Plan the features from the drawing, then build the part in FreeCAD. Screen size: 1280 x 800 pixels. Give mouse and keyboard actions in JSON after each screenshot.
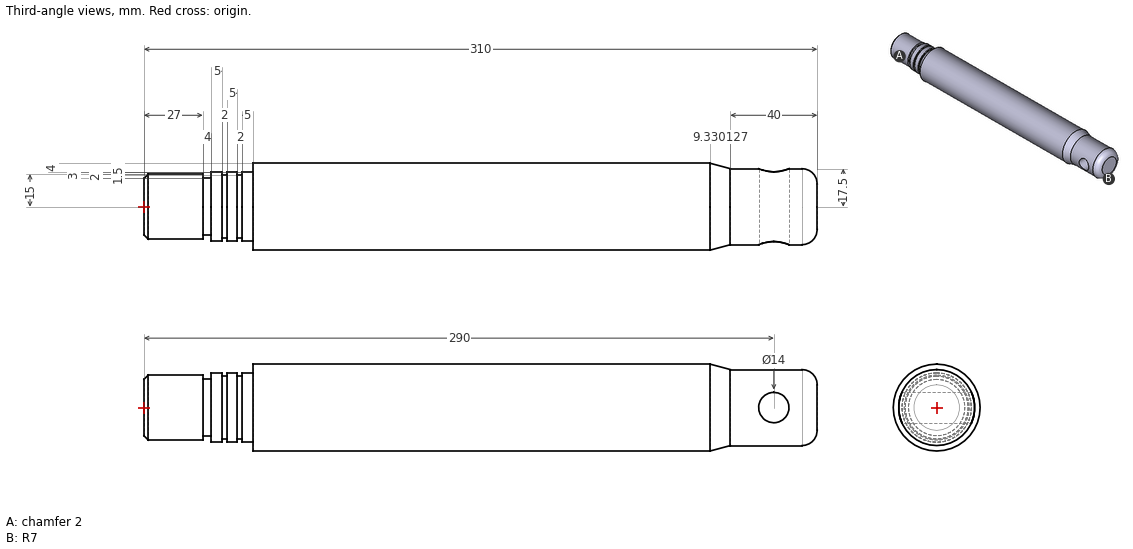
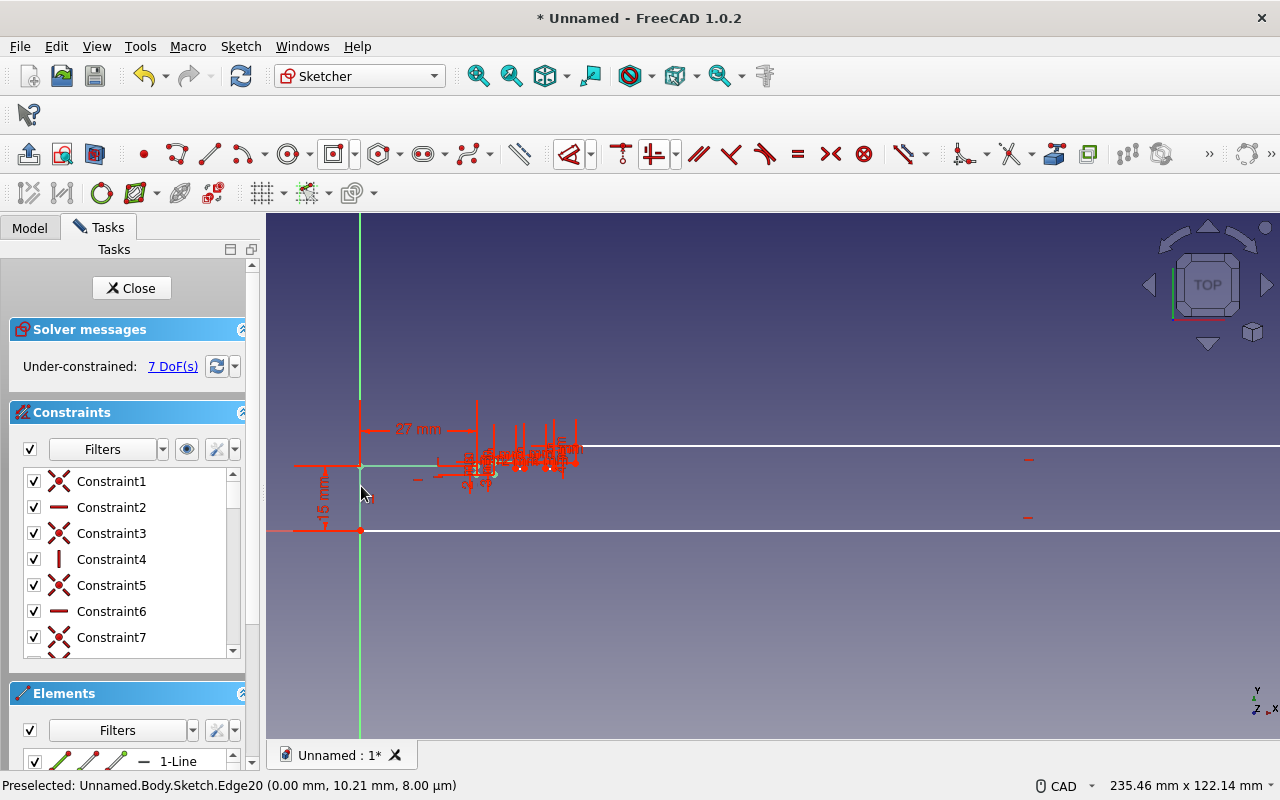
{"action": "left_click", "coordinate": [761, 531]}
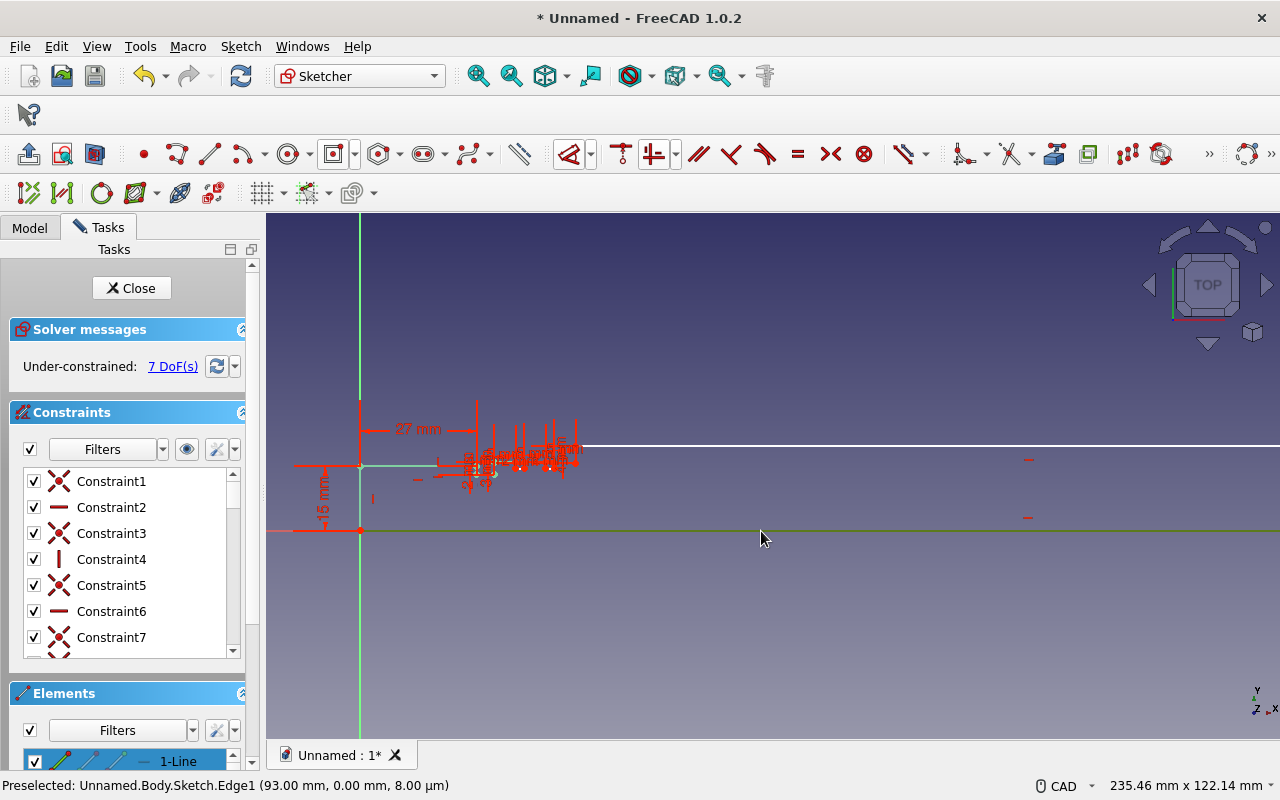
{"action": "left_click", "coordinate": [590, 154]}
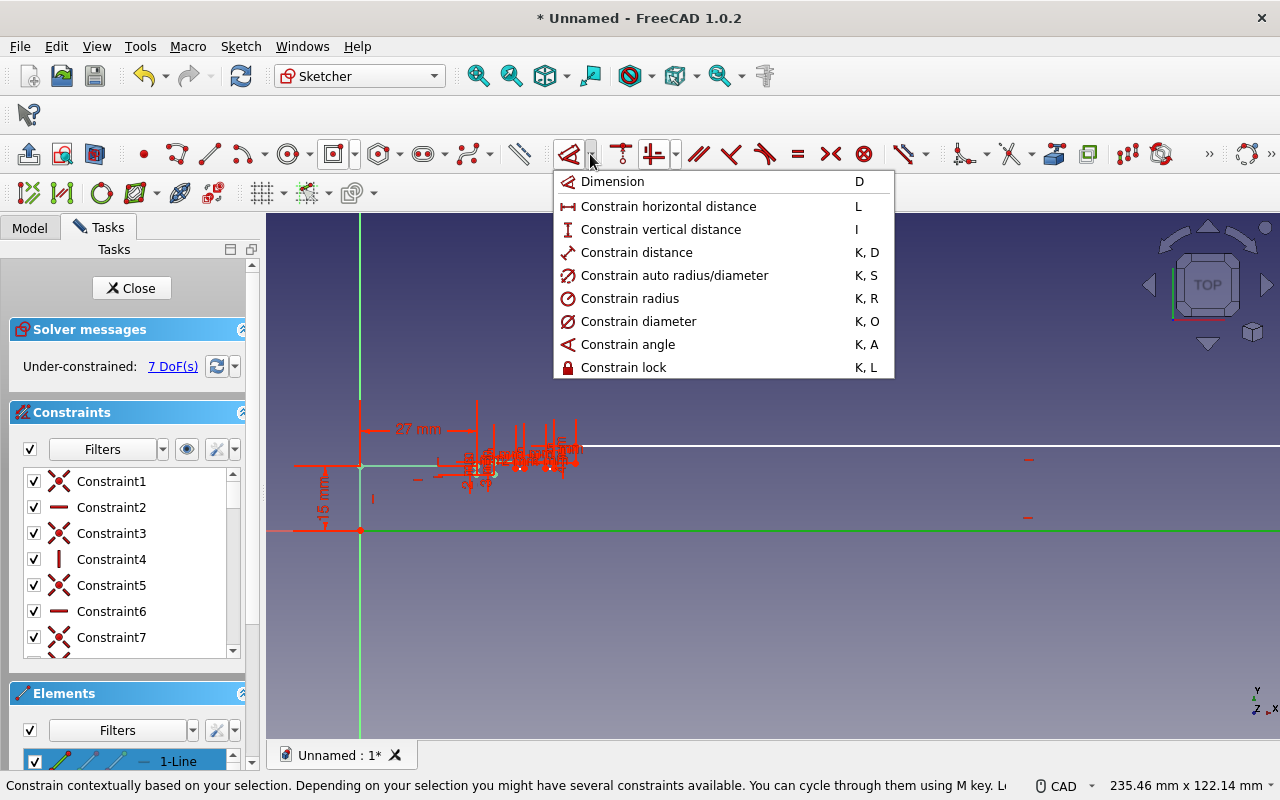
{"action": "left_click", "coordinate": [724, 206]}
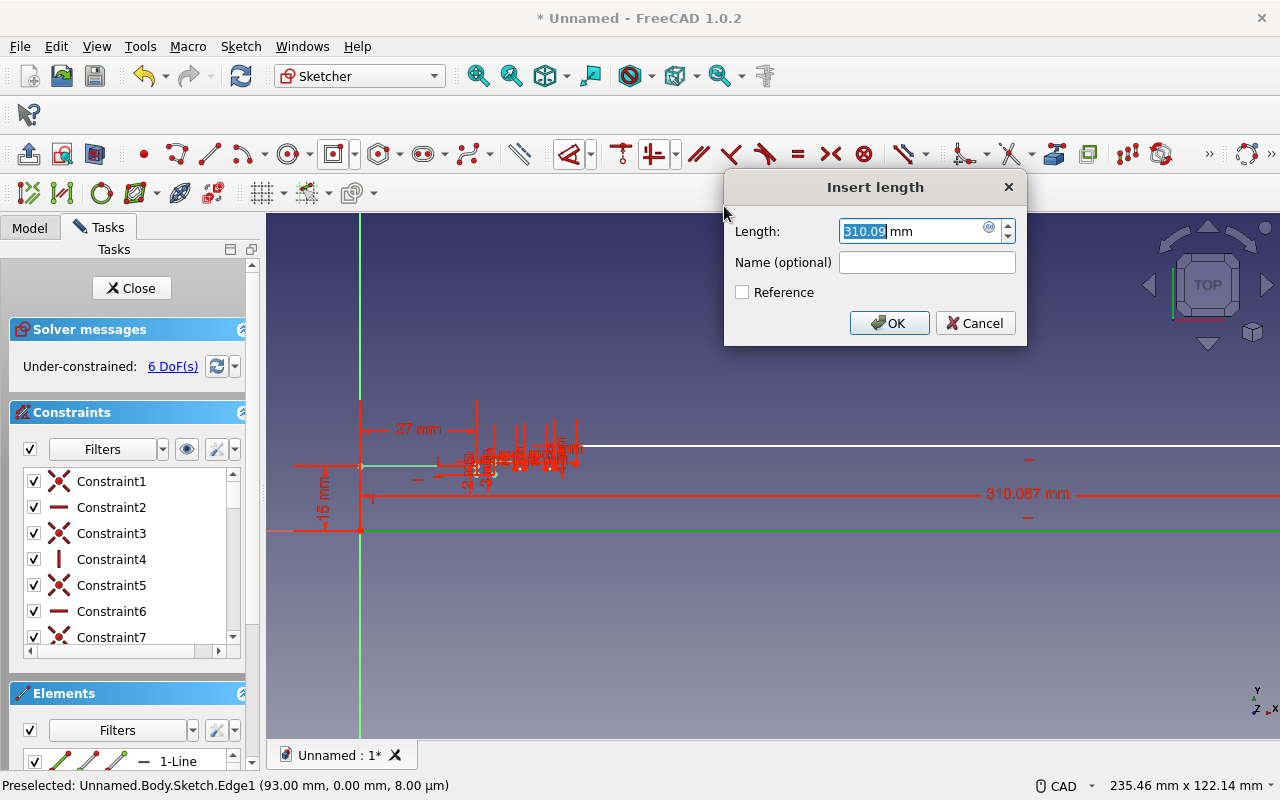
{"action": "type", "text": "310"}
{"action": "key", "text": "Return"}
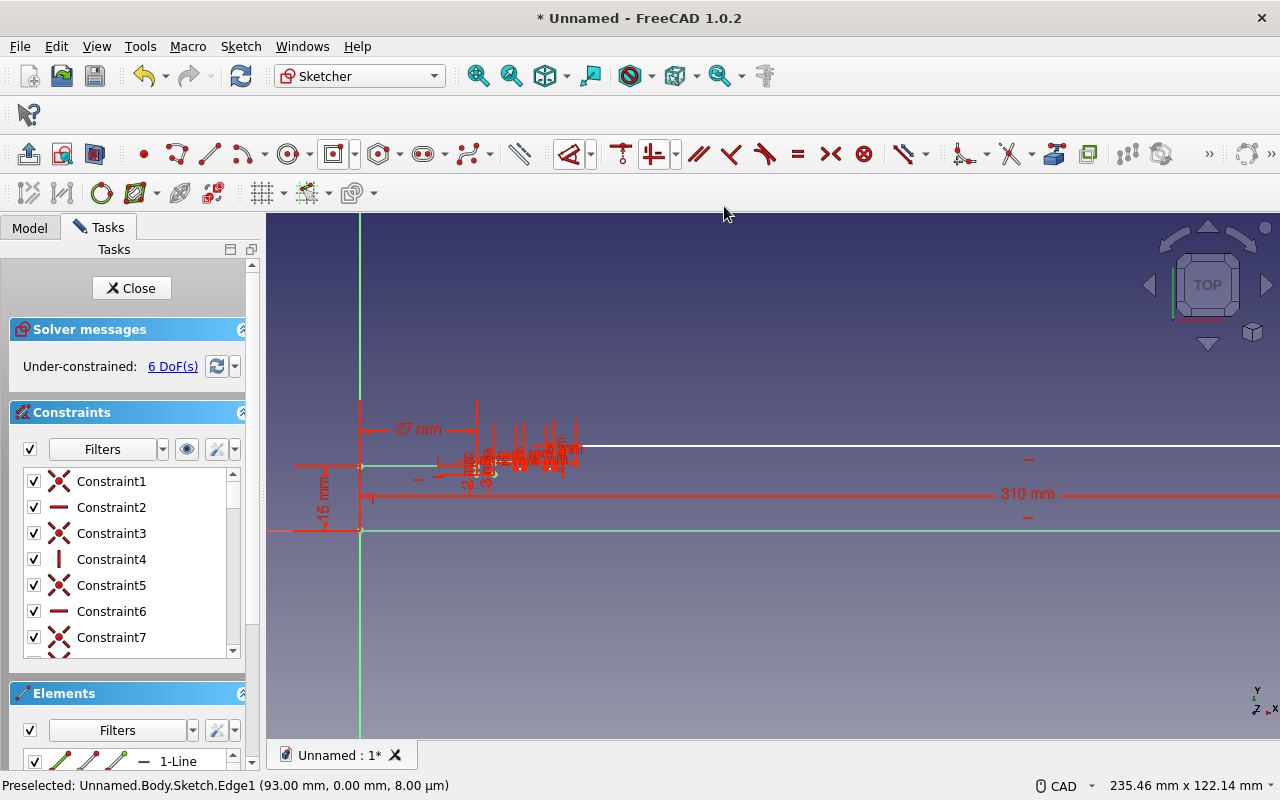
{"action": "scroll", "coordinate": [554, 466], "scroll_direction": "up", "scroll_amount": 10}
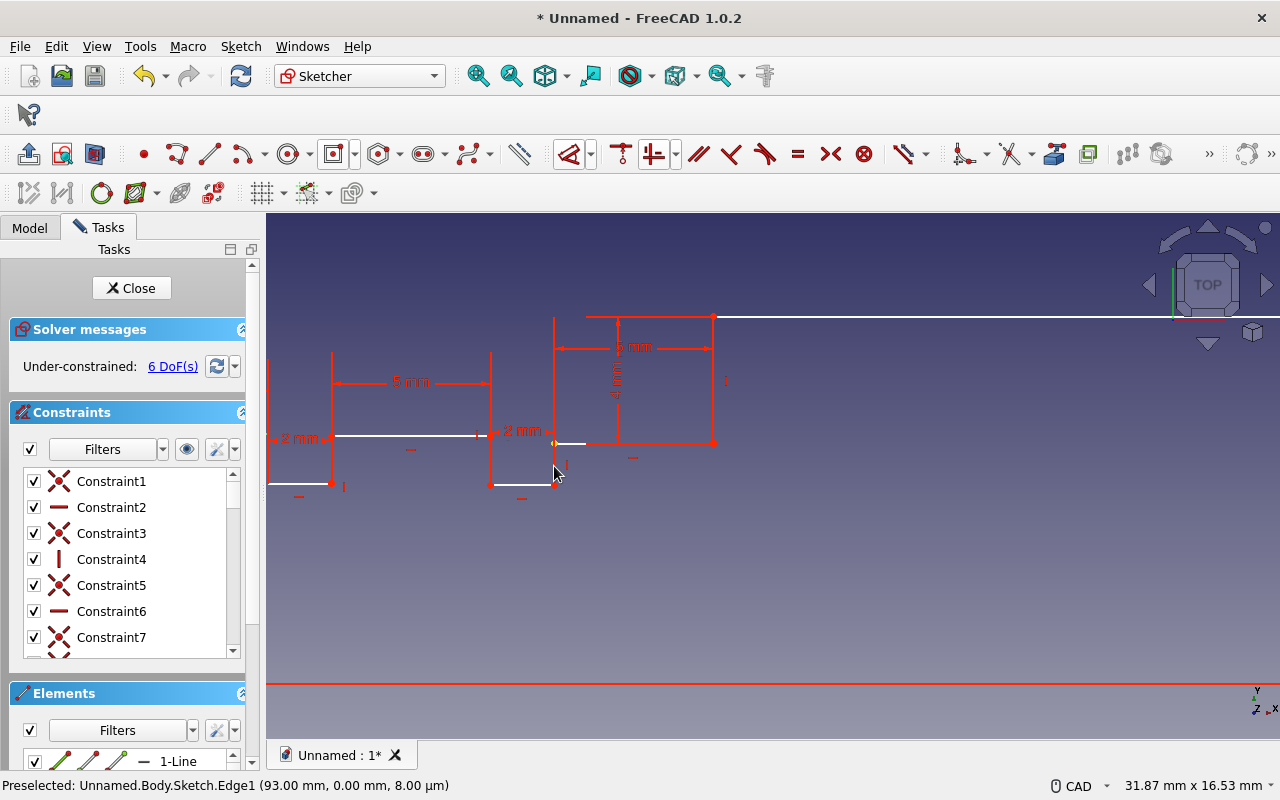
{"action": "left_click", "coordinate": [554, 464]}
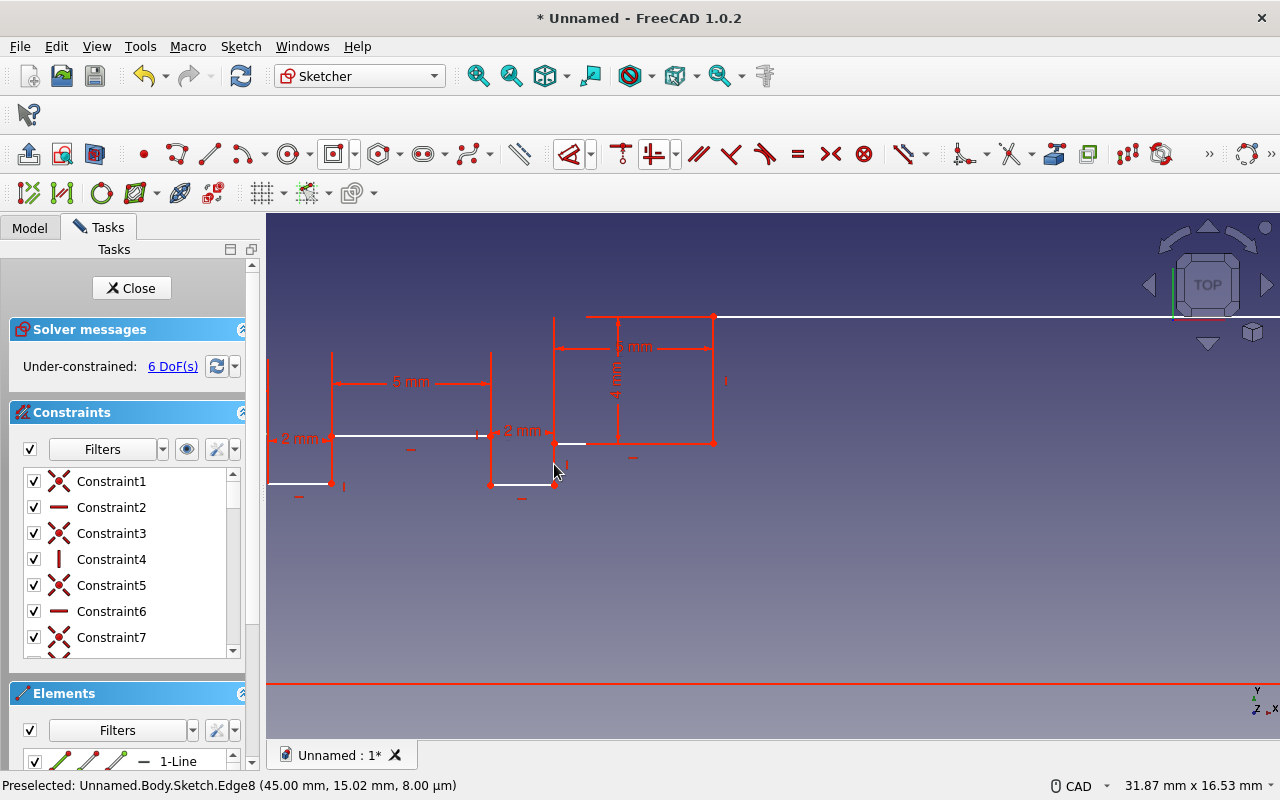
{"action": "key", "text": "i"}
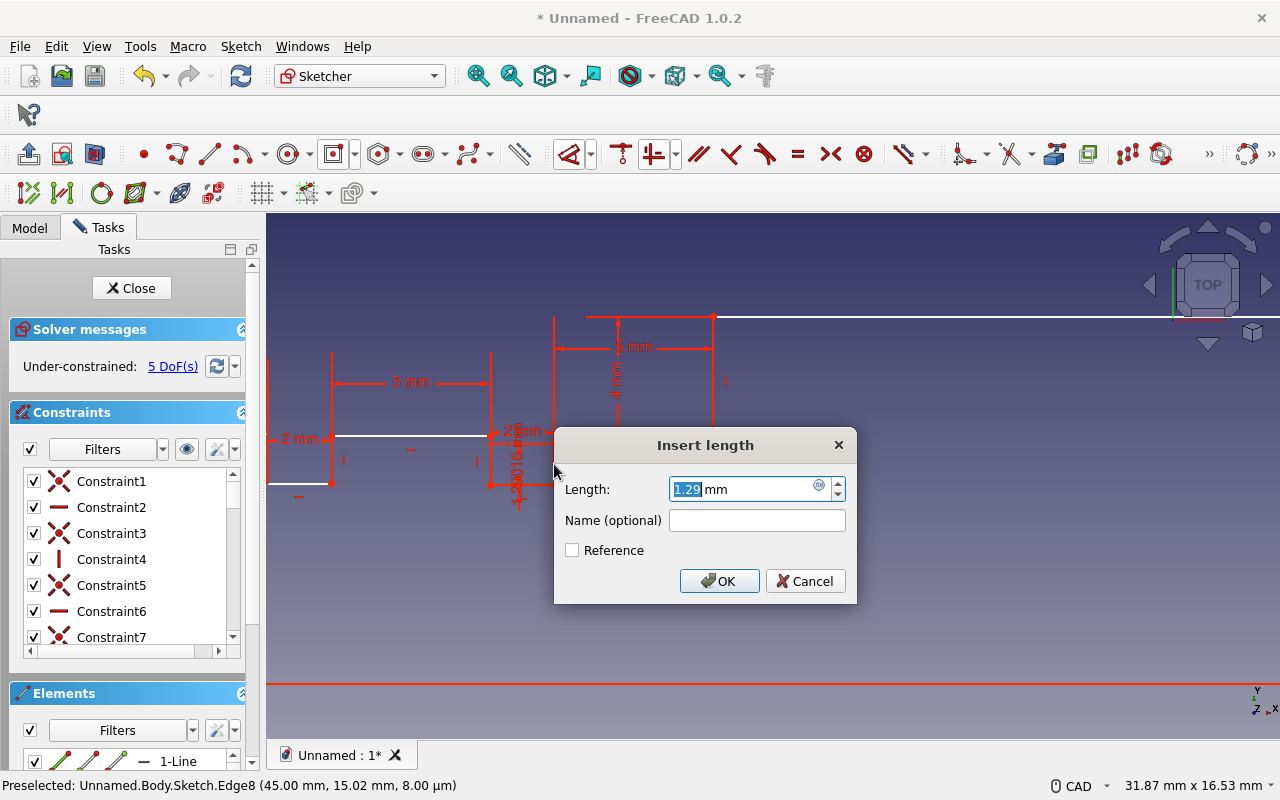
{"action": "type", "text": "1.5"}
{"action": "key", "text": "Return"}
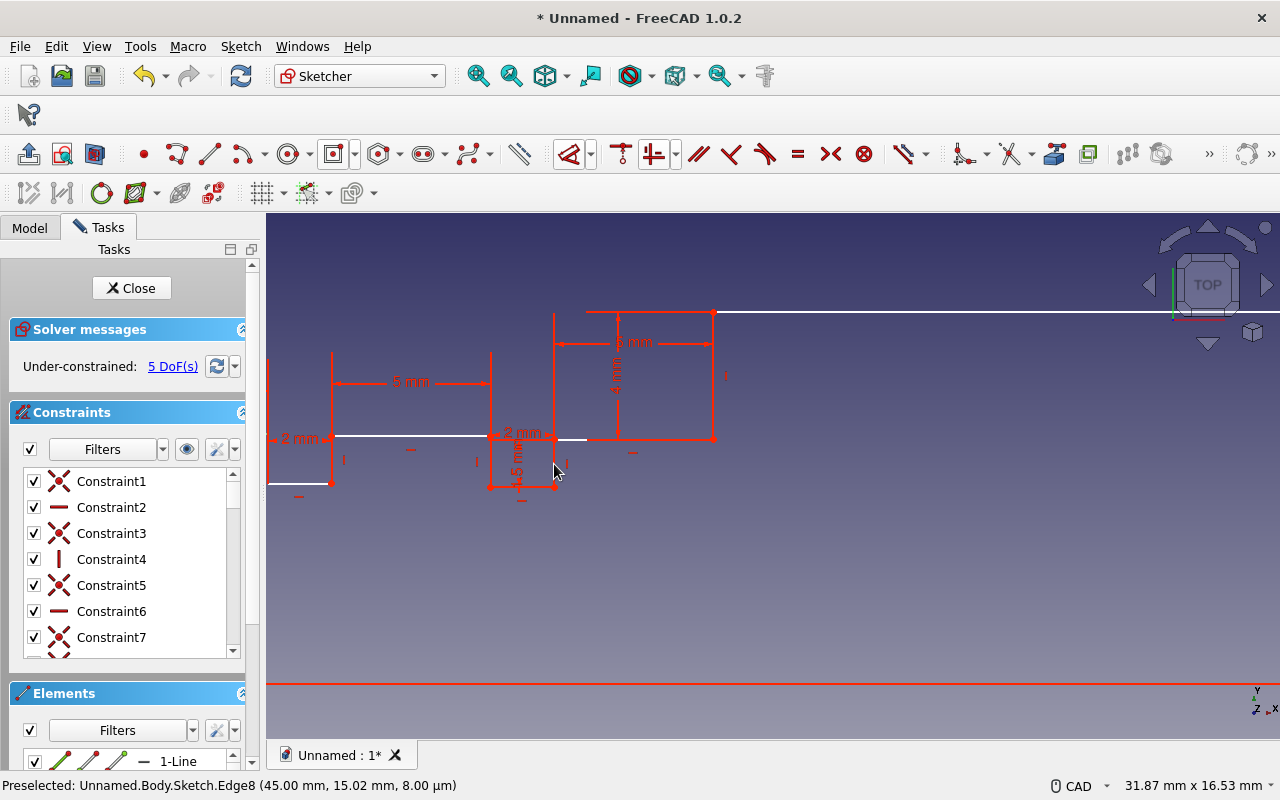
{"action": "left_click", "coordinate": [491, 472]}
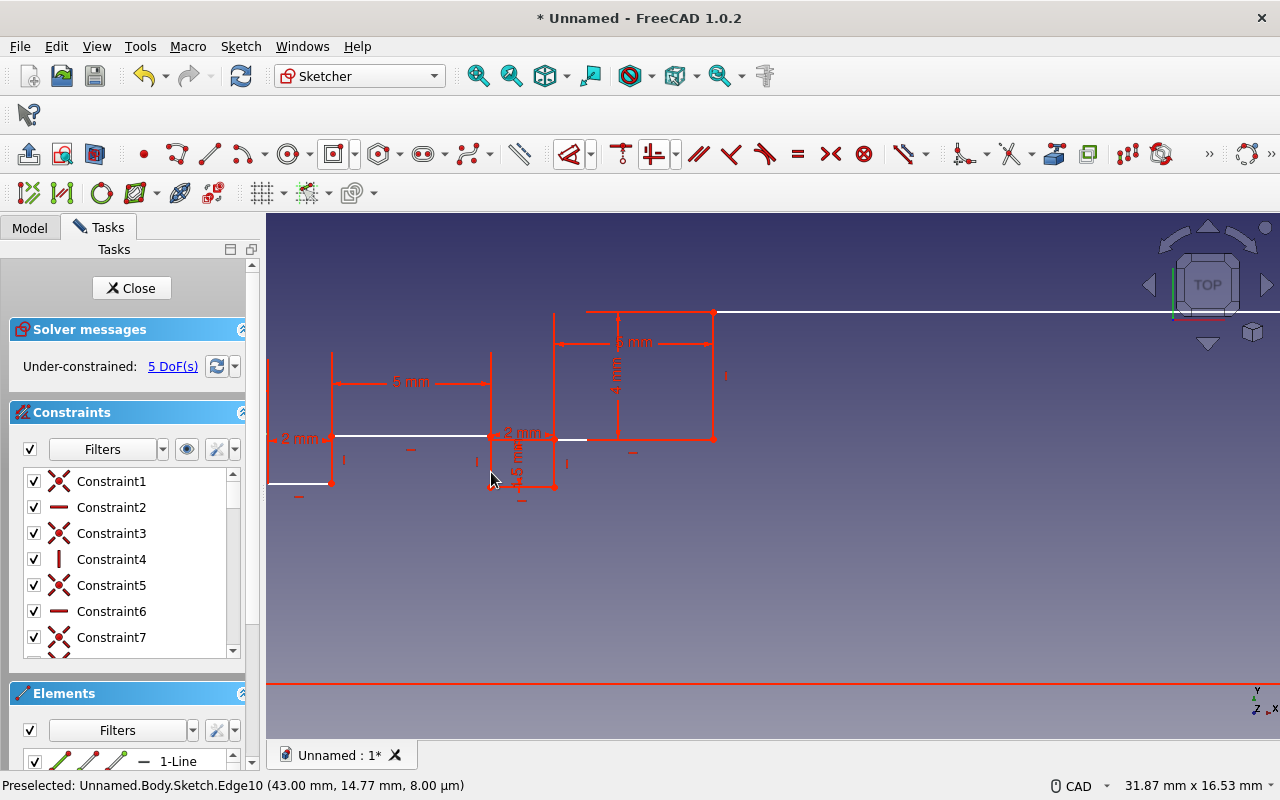
{"action": "key", "text": "i"}